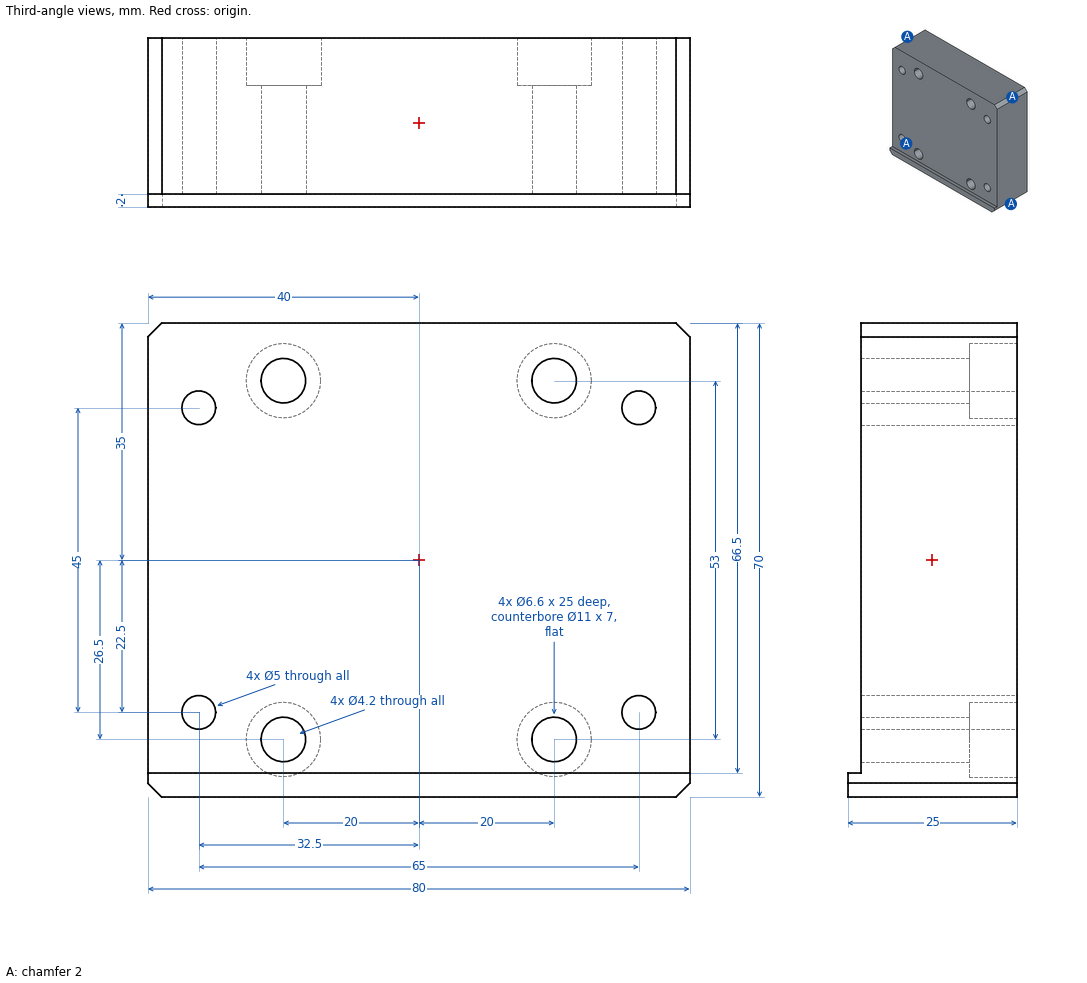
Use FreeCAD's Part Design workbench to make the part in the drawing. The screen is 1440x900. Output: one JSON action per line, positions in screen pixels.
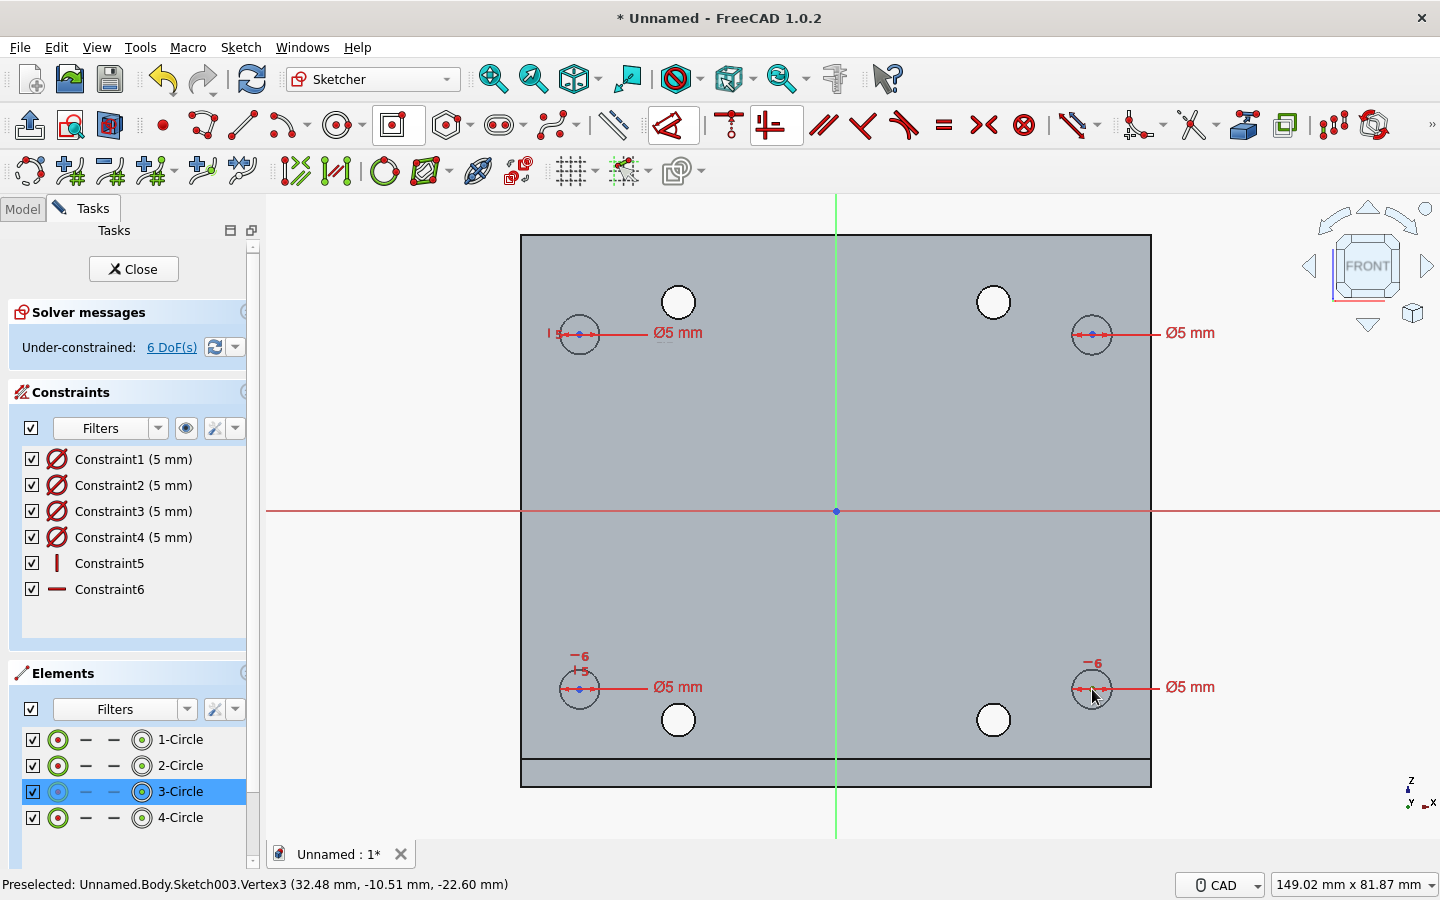
{"action": "left_click", "coordinate": [1092, 335]}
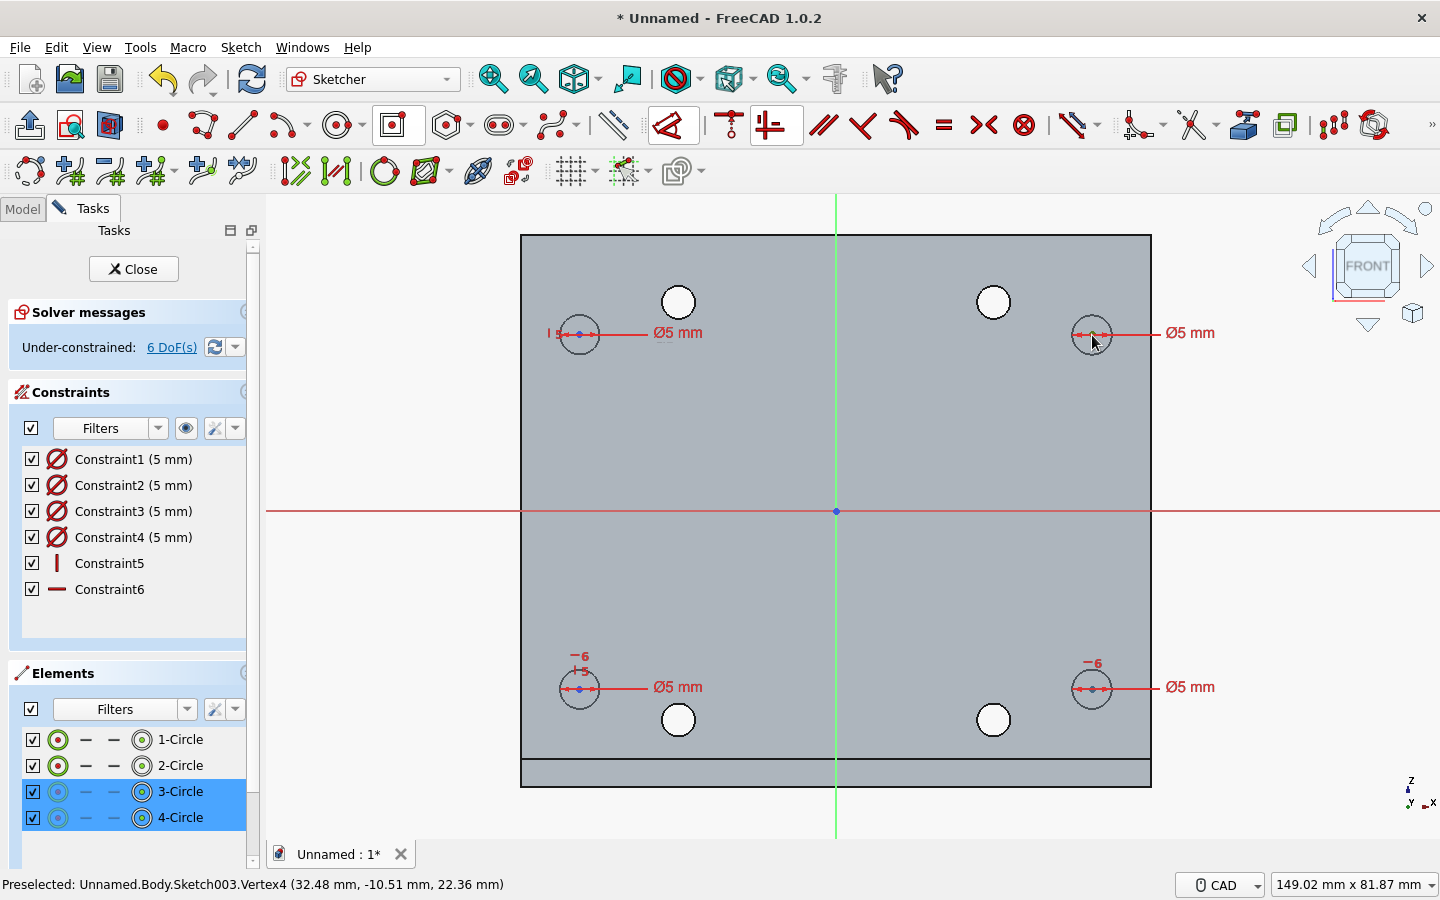
{"action": "key", "text": "v"}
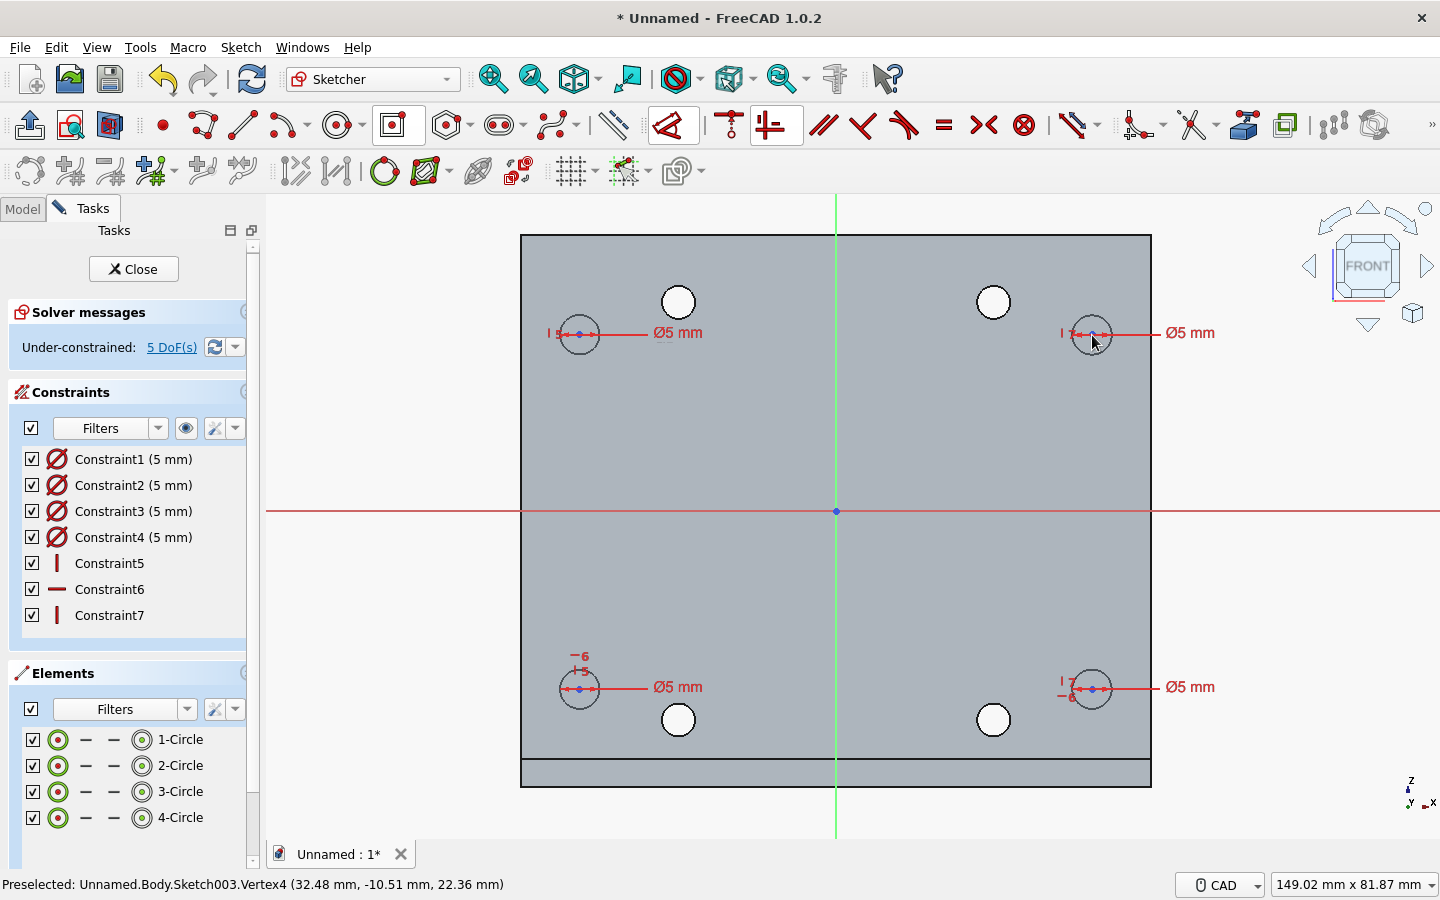
{"action": "left_click", "coordinate": [580, 335]}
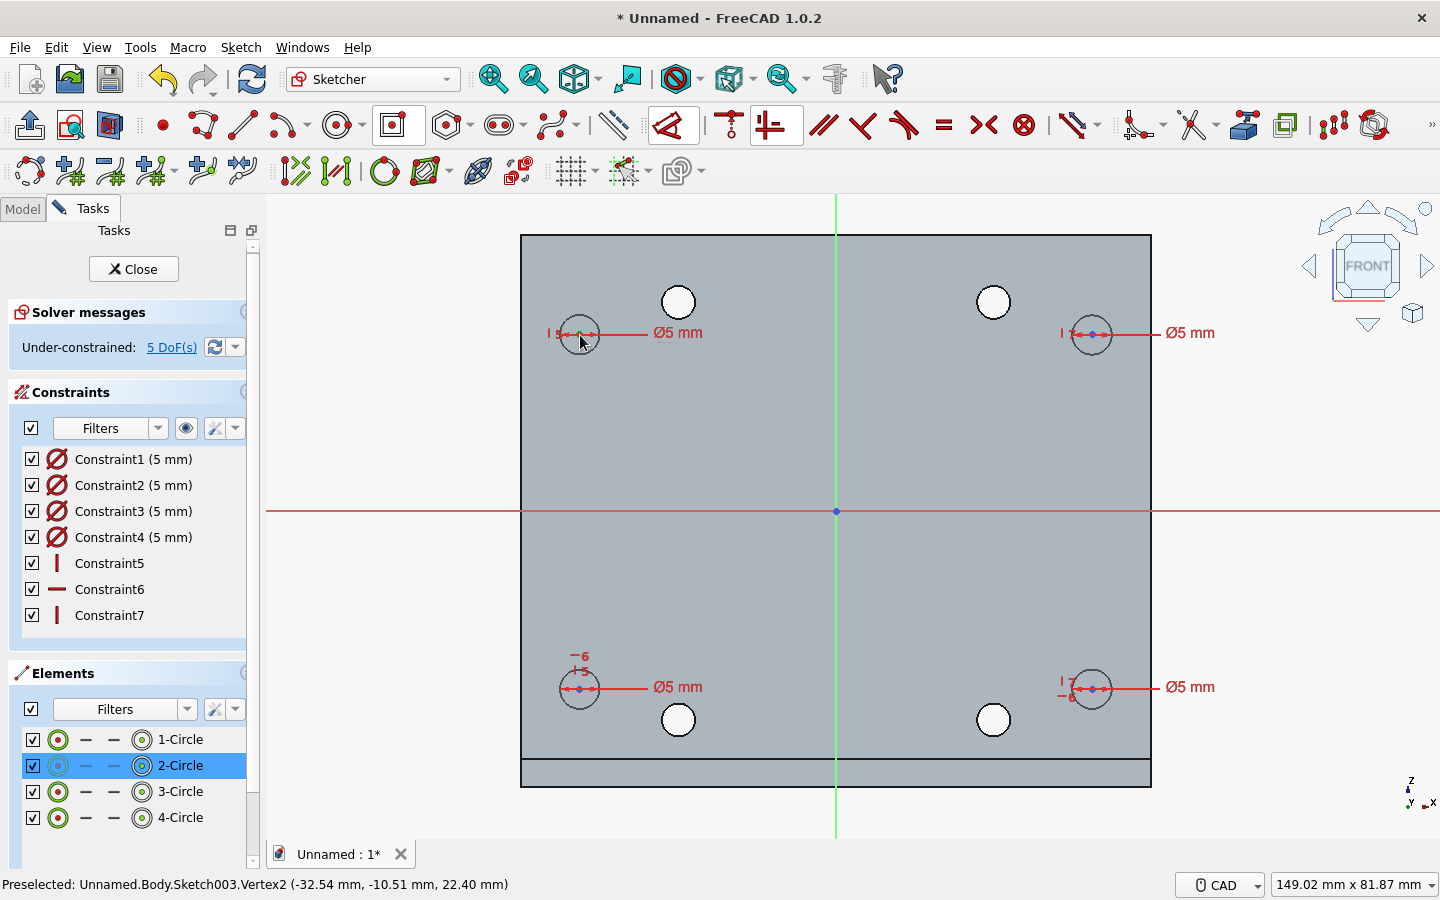
{"action": "left_click", "coordinate": [1092, 335]}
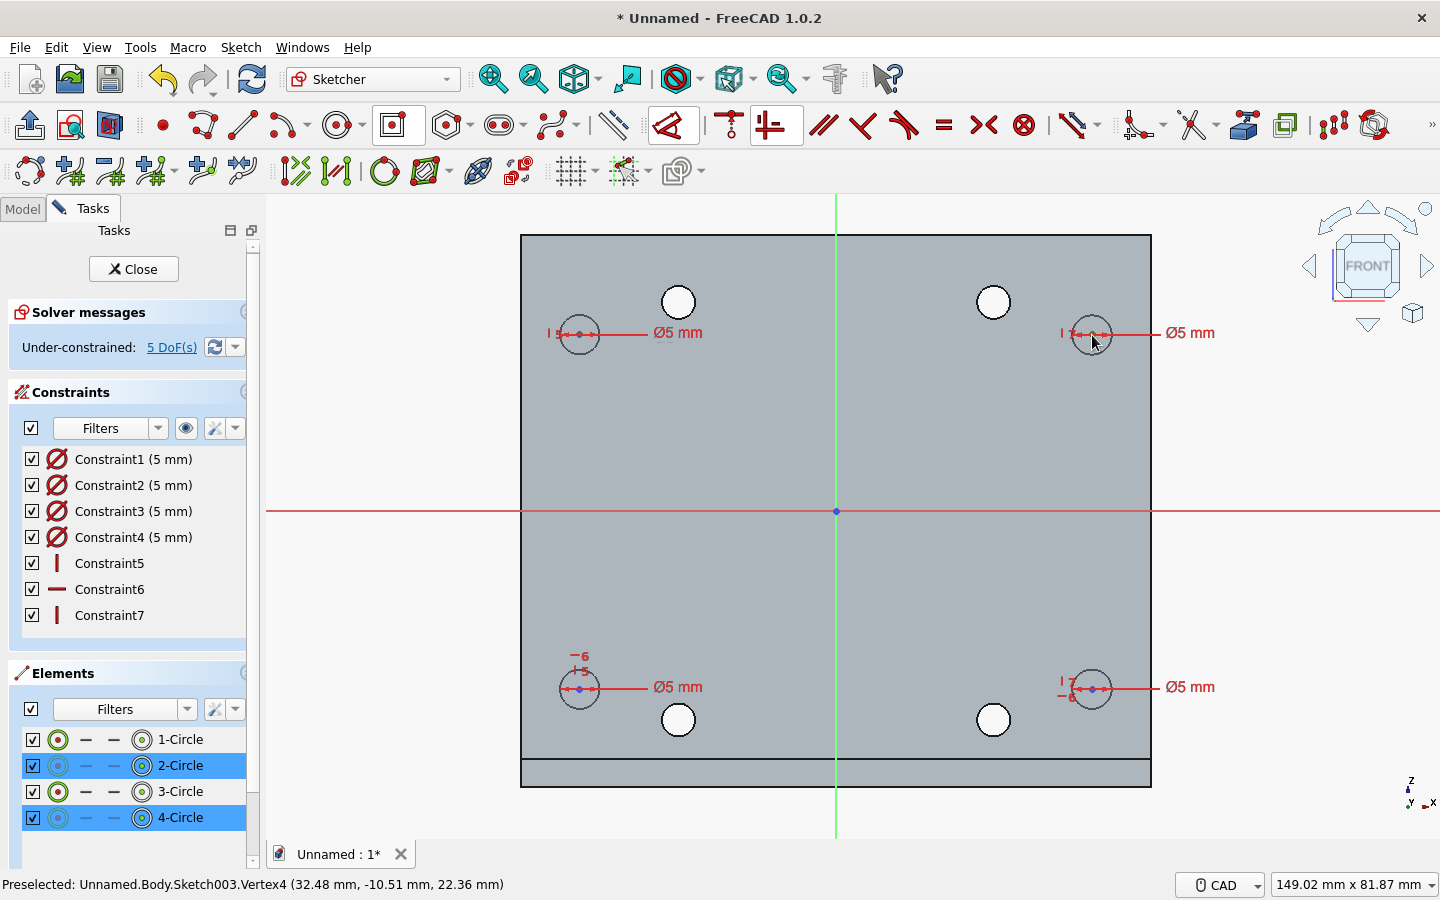
{"action": "key", "text": "h"}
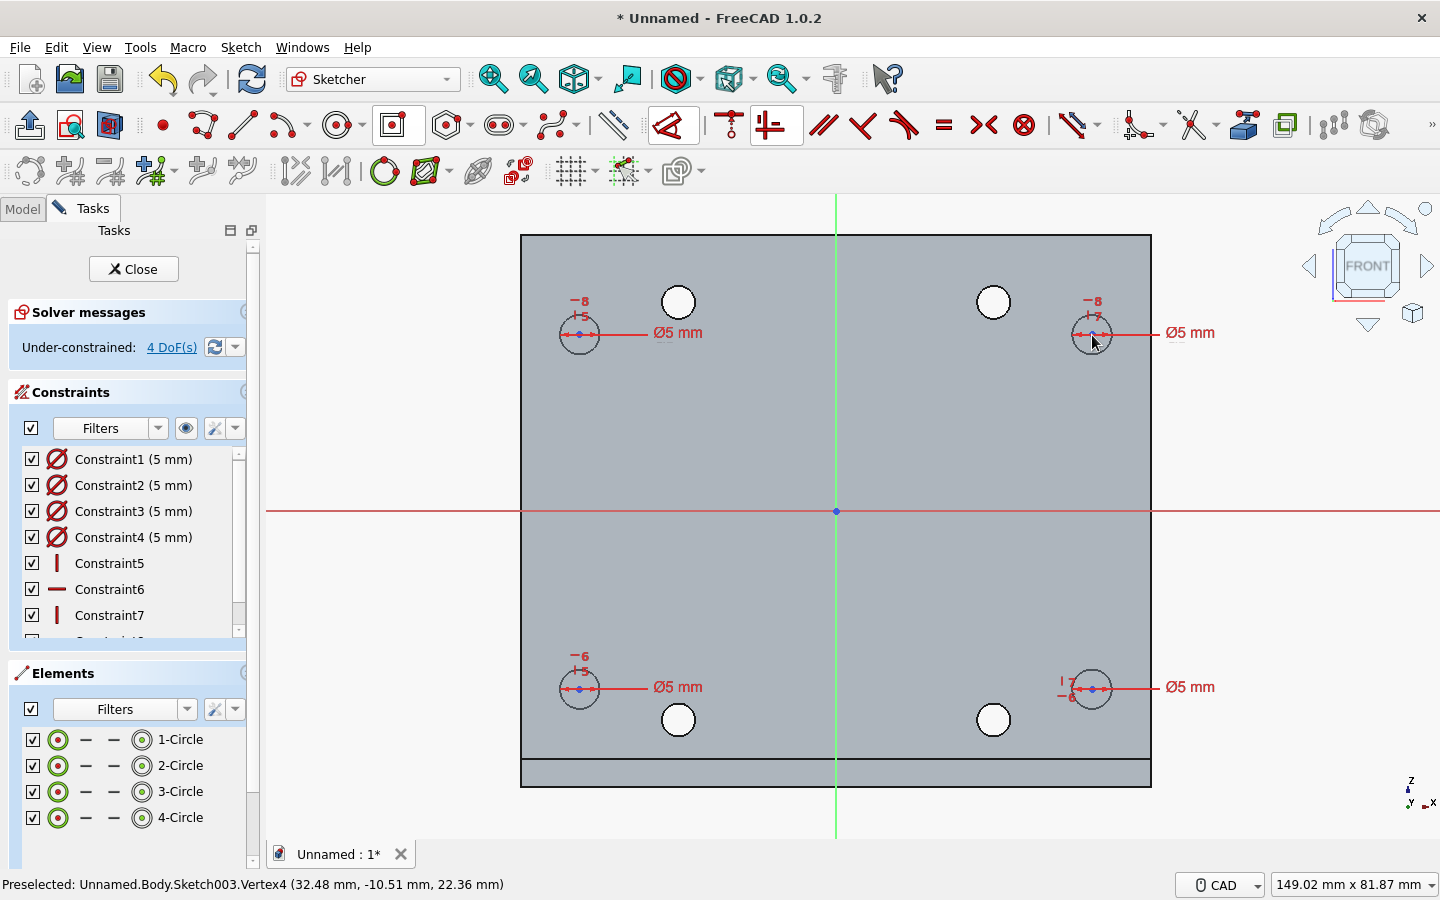
{"action": "left_click", "coordinate": [580, 689]}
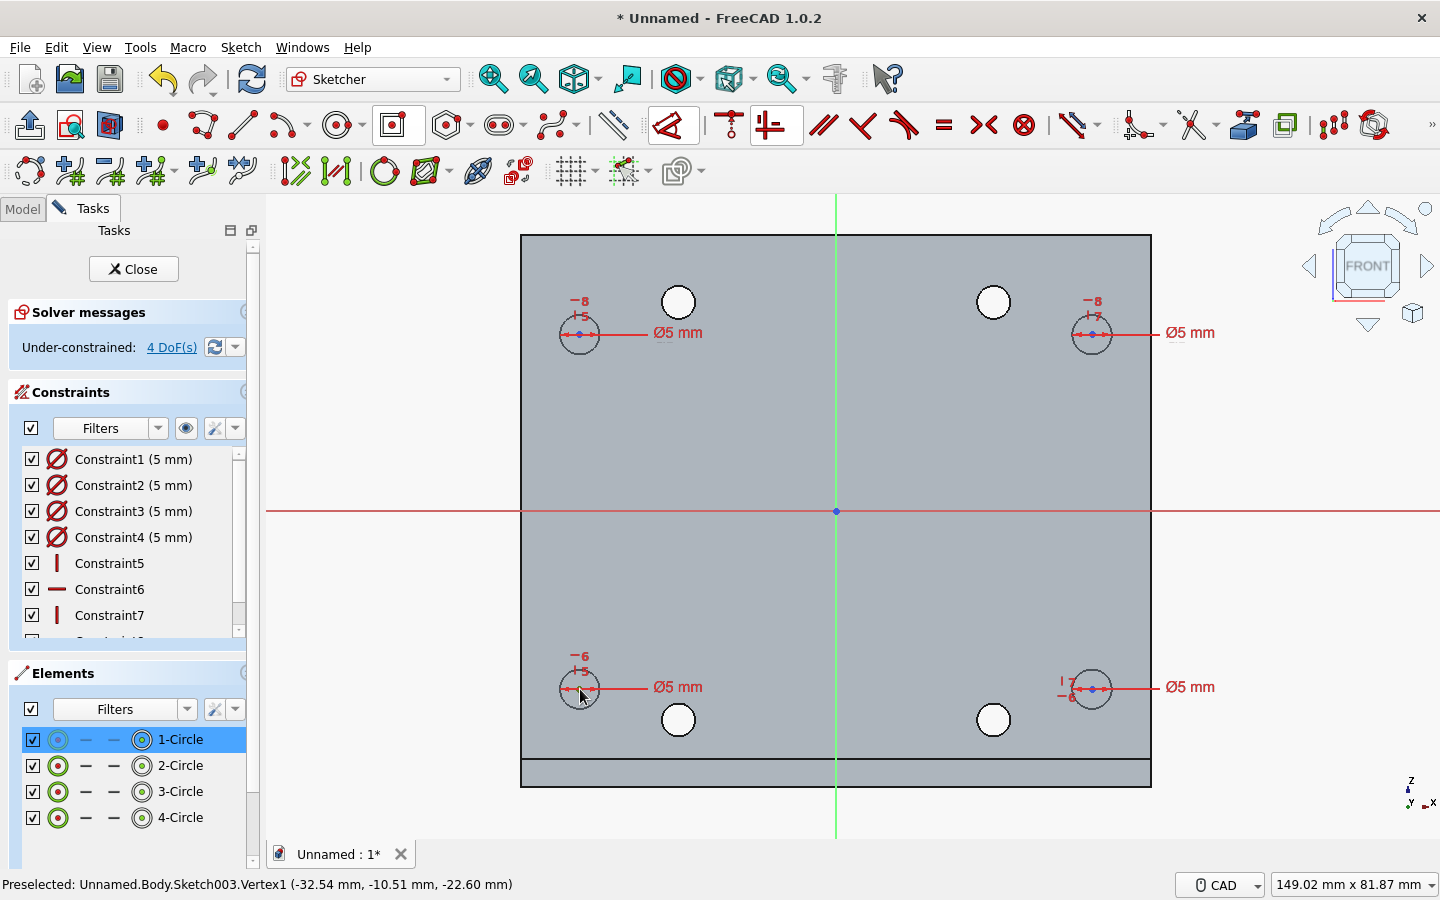
{"action": "left_click", "coordinate": [580, 335]}